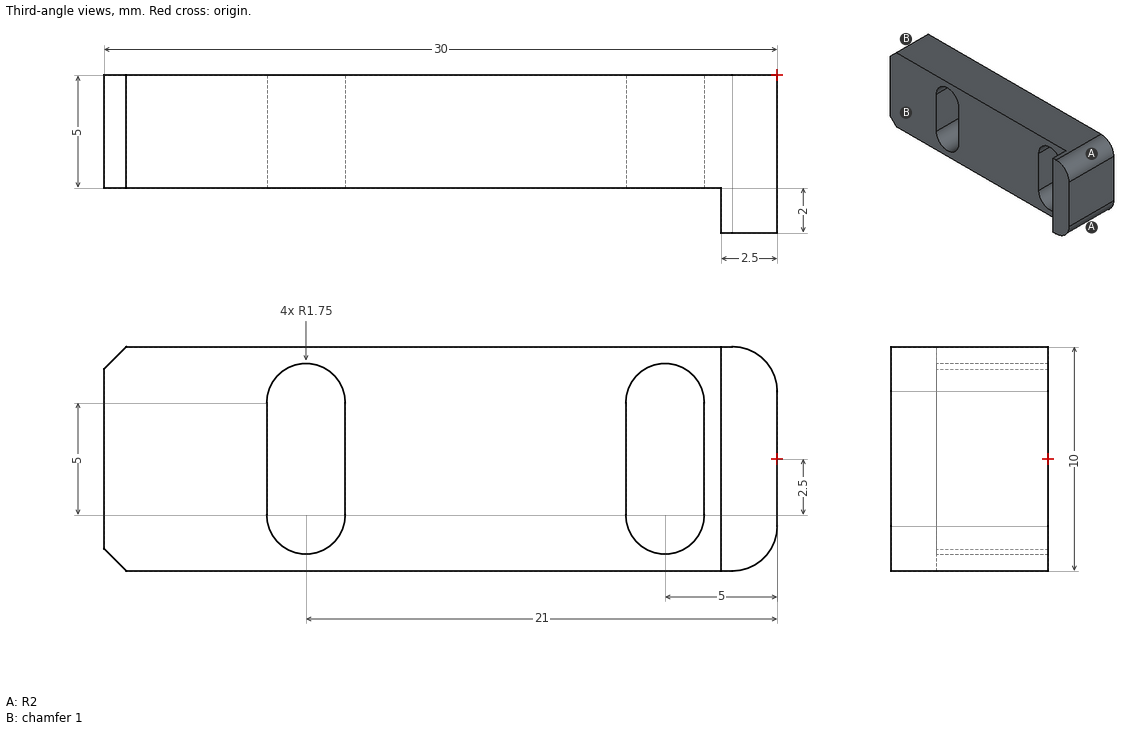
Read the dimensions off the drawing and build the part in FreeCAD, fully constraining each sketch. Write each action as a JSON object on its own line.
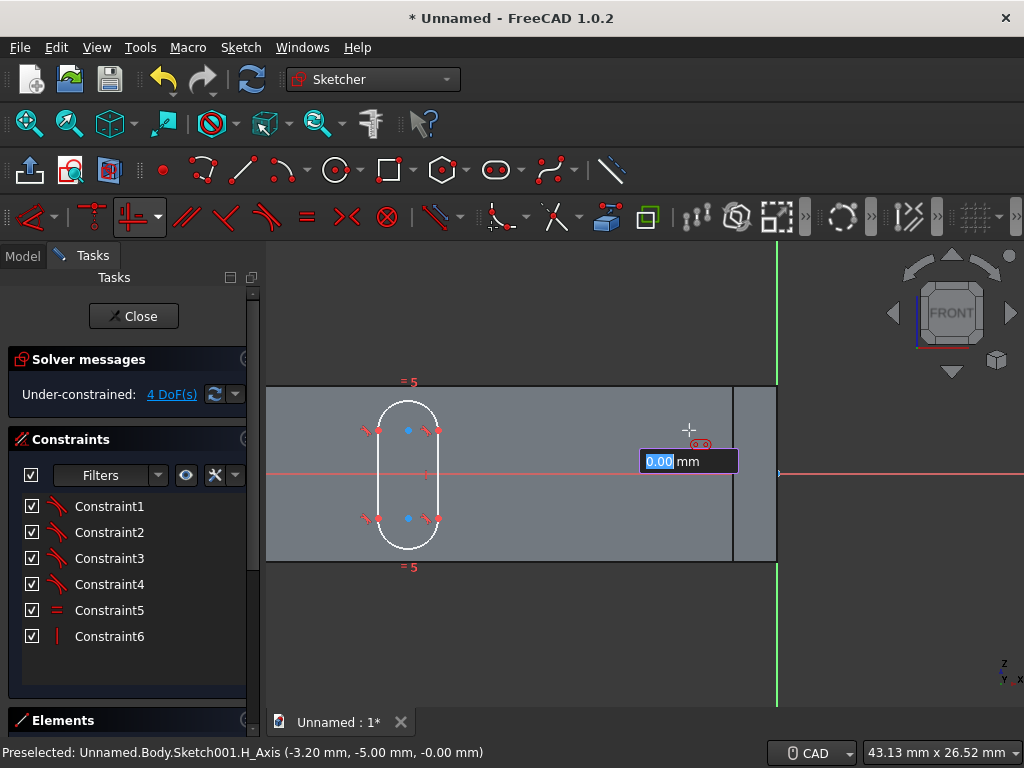
{"action": "left_click", "coordinate": [719, 487]}
{"action": "key", "text": "Escape"}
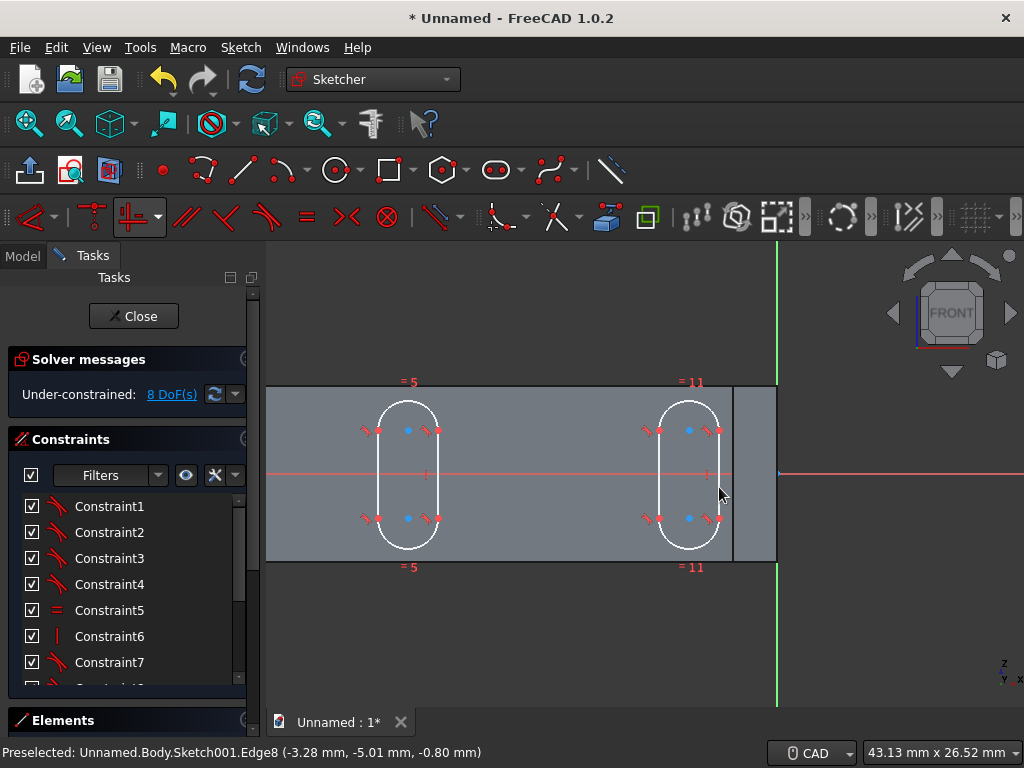
{"action": "left_click", "coordinate": [390, 543]}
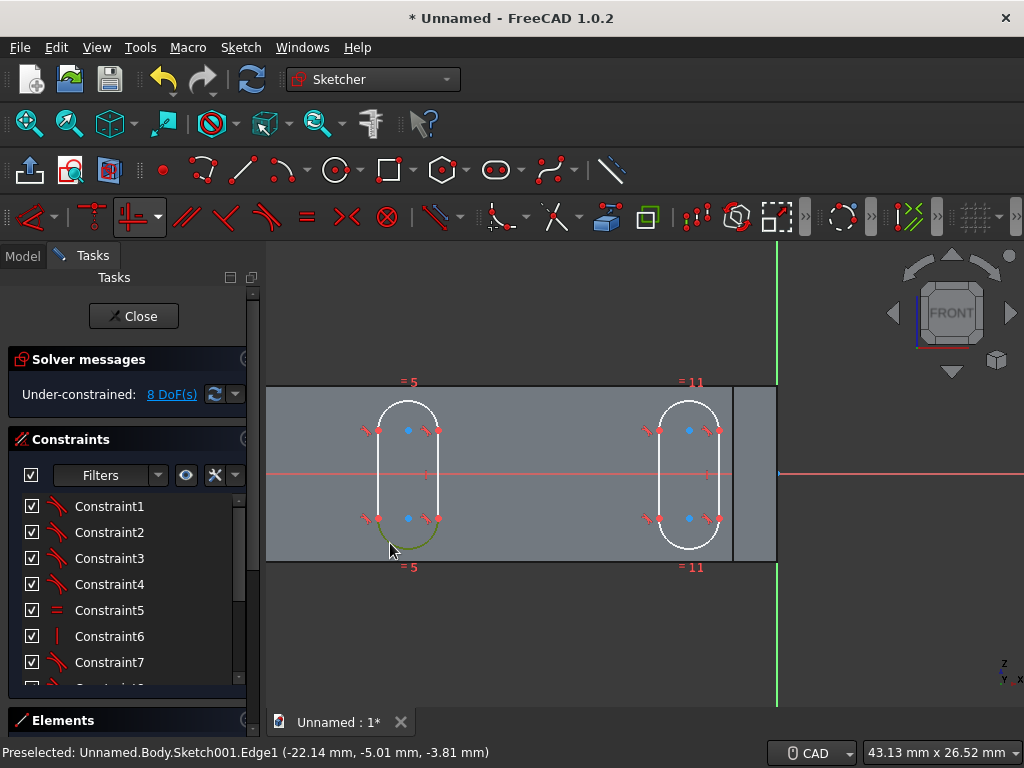
{"action": "left_click", "coordinate": [671, 543]}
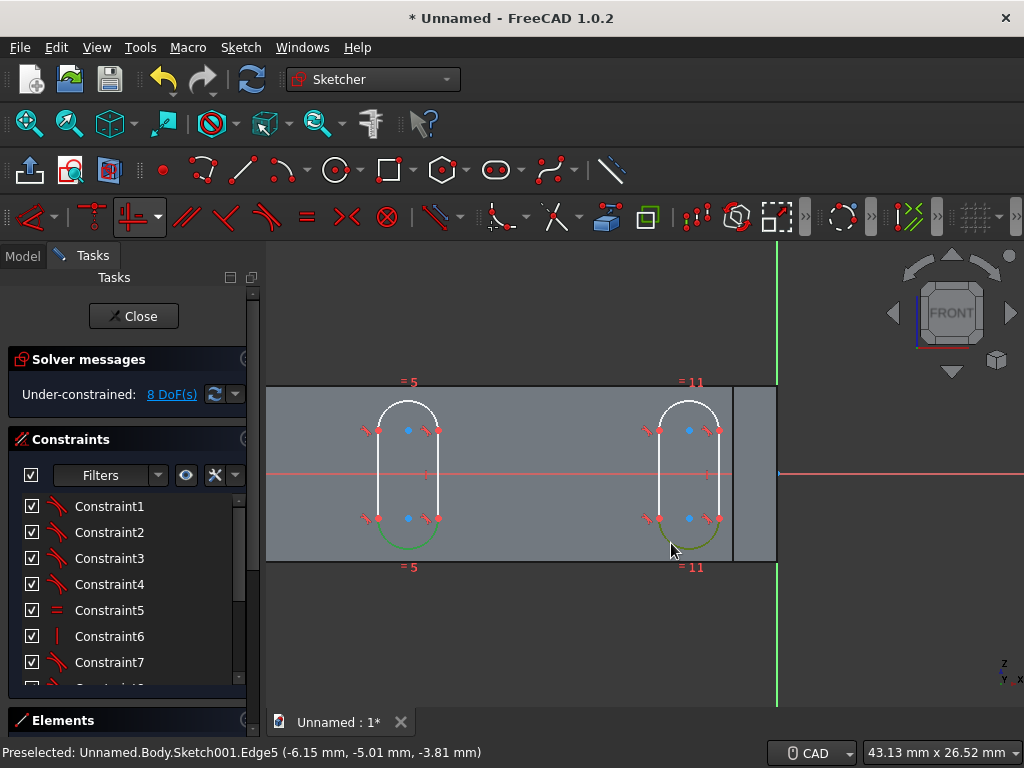
{"action": "left_click", "coordinate": [308, 218]}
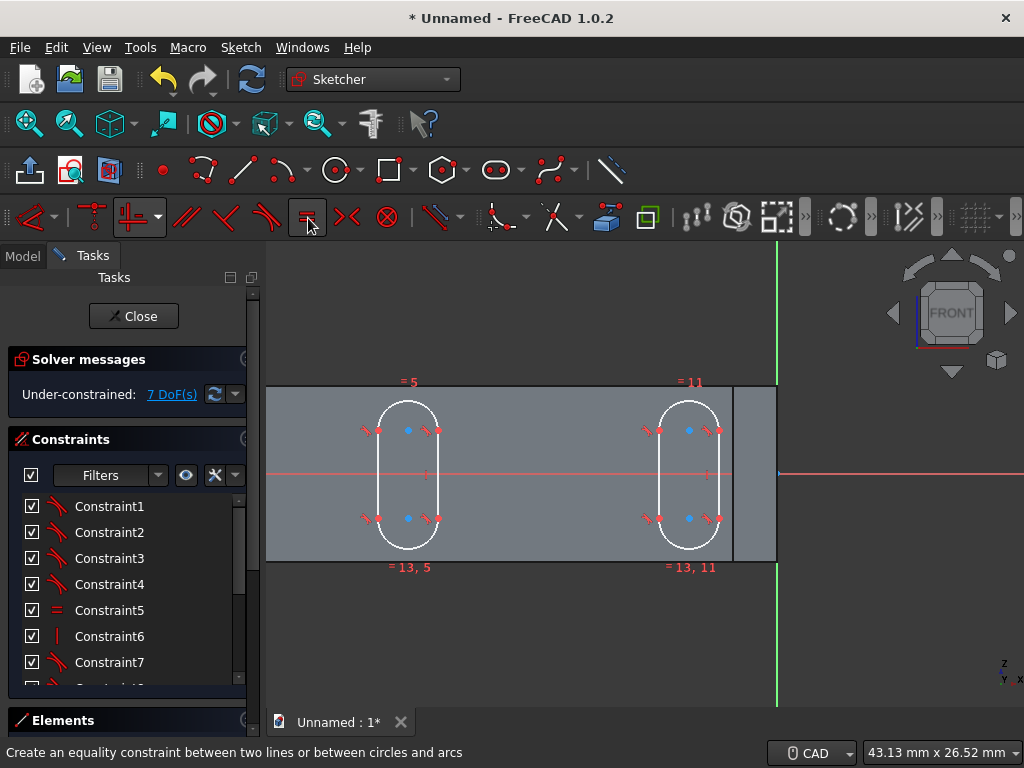
{"action": "scroll", "coordinate": [390, 543], "scroll_direction": "up", "scroll_amount": 2}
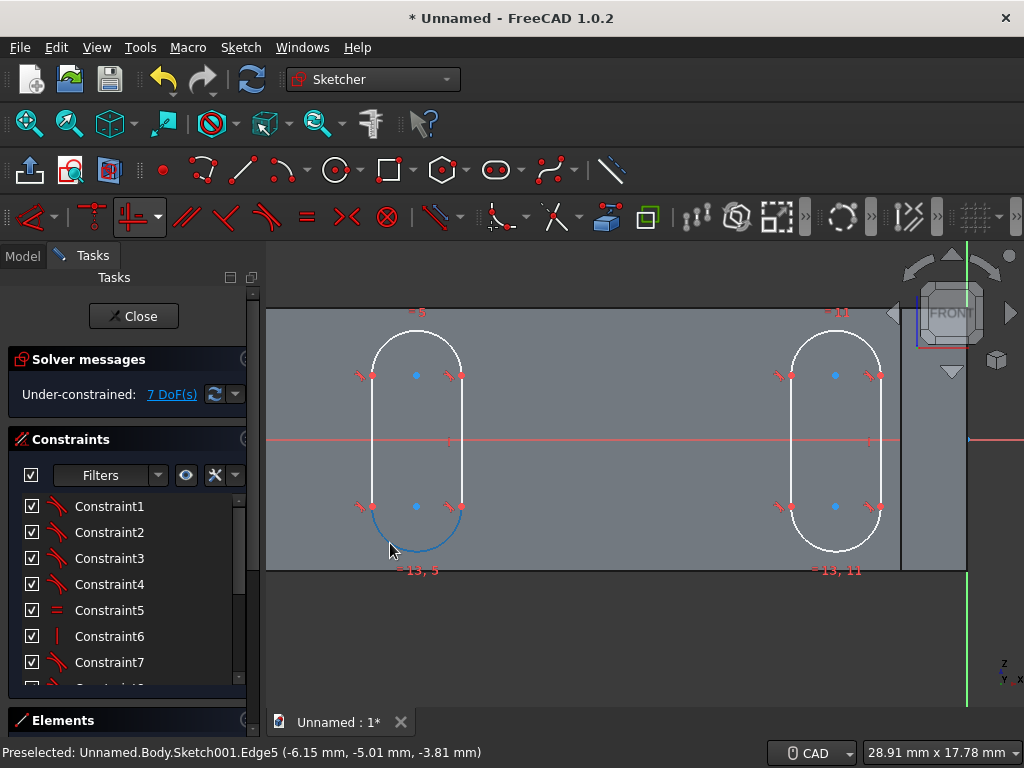
{"action": "left_click", "coordinate": [390, 543]}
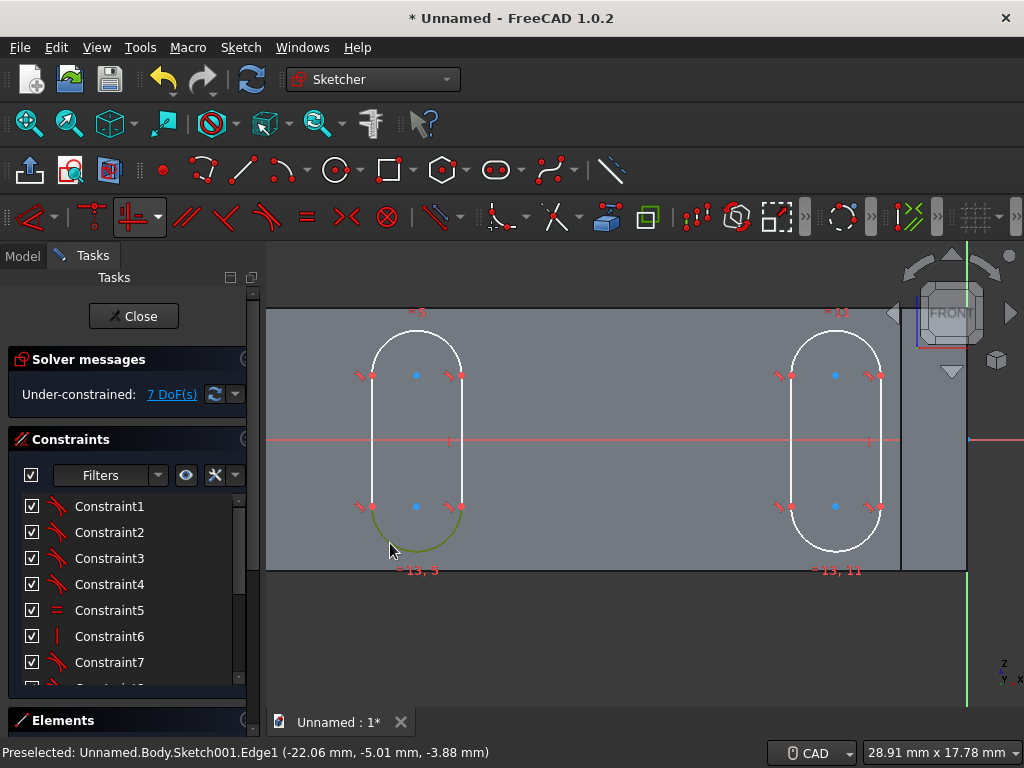
{"action": "key", "text": "k r"}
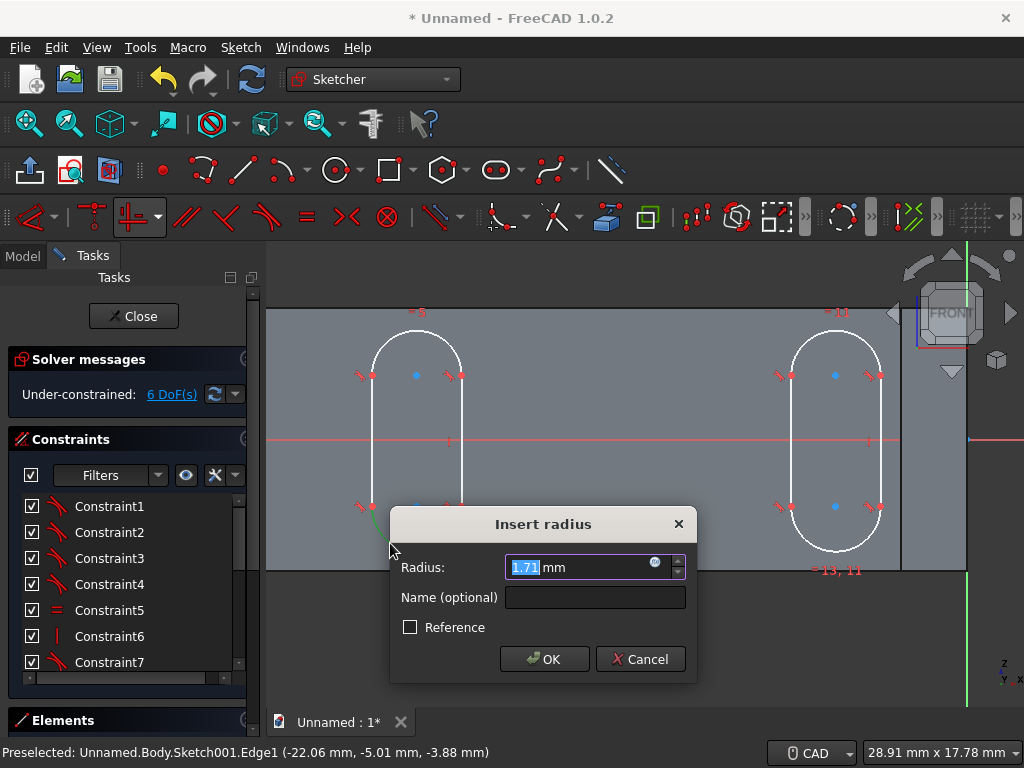
{"action": "type", "text": "1.75"}
{"action": "key", "text": "Return"}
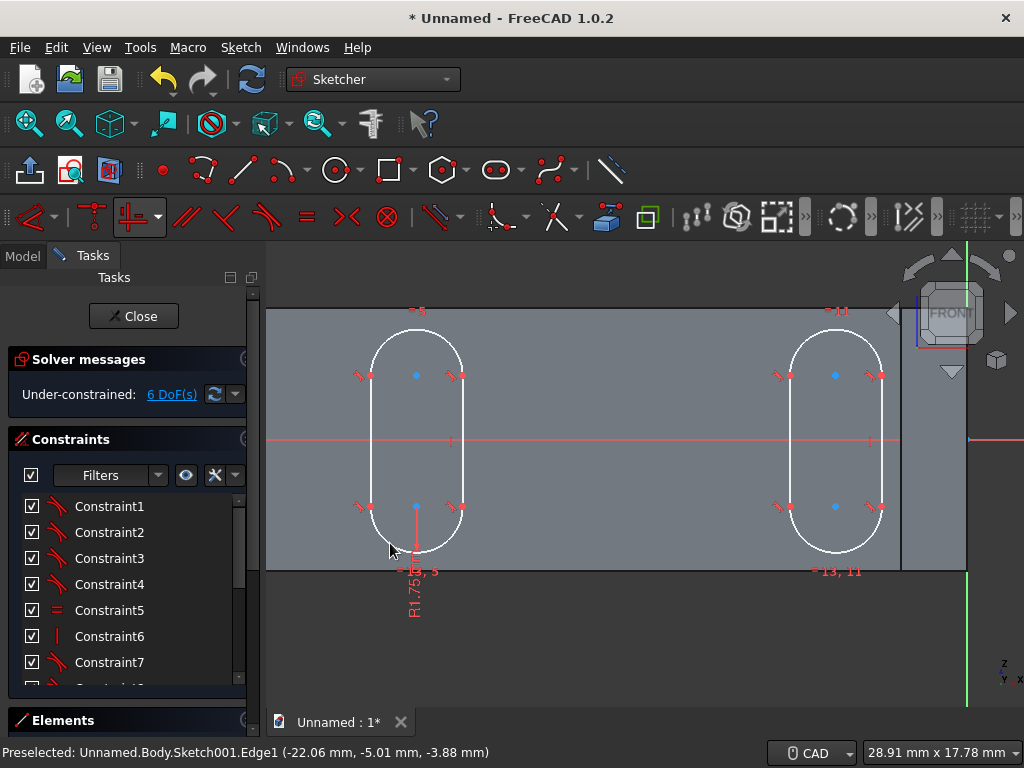
{"action": "left_click", "coordinate": [371, 467]}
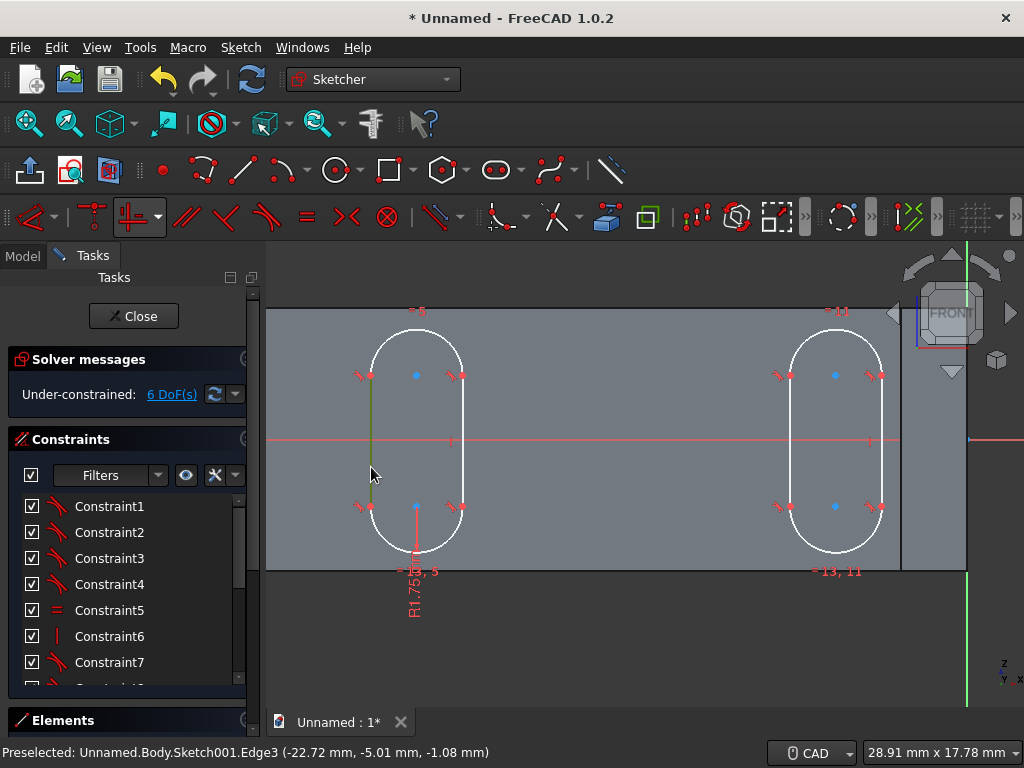
{"action": "key", "text": "i"}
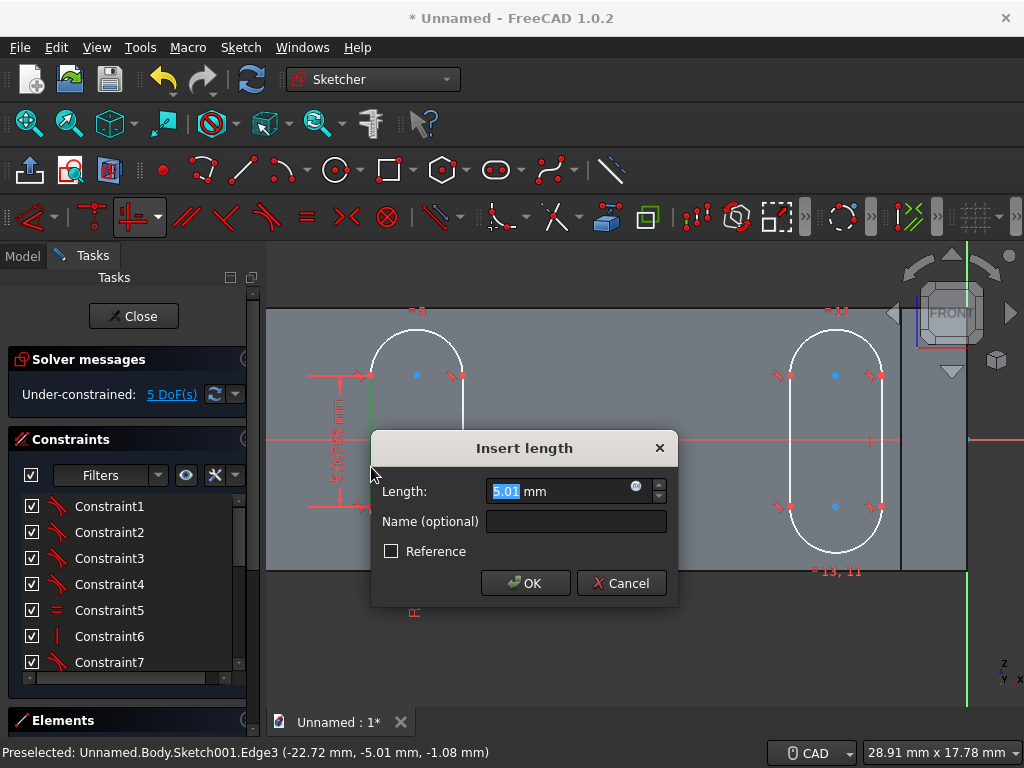
{"action": "type", "text": "5"}
{"action": "key", "text": "Return"}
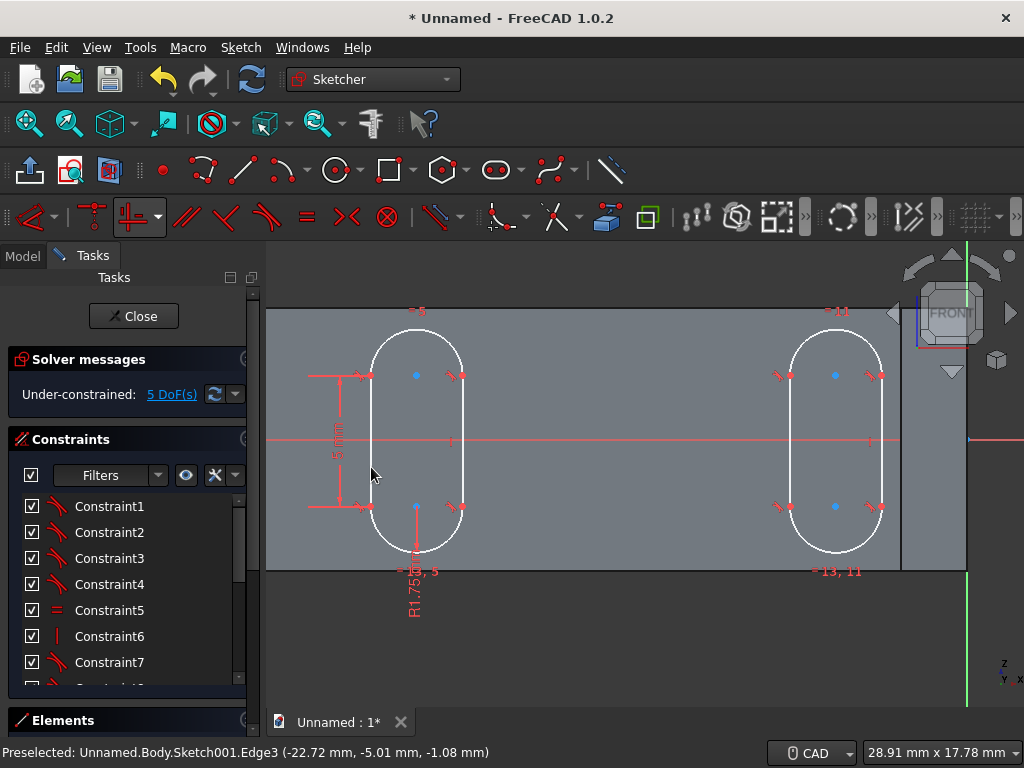
{"action": "left_click", "coordinate": [790, 467]}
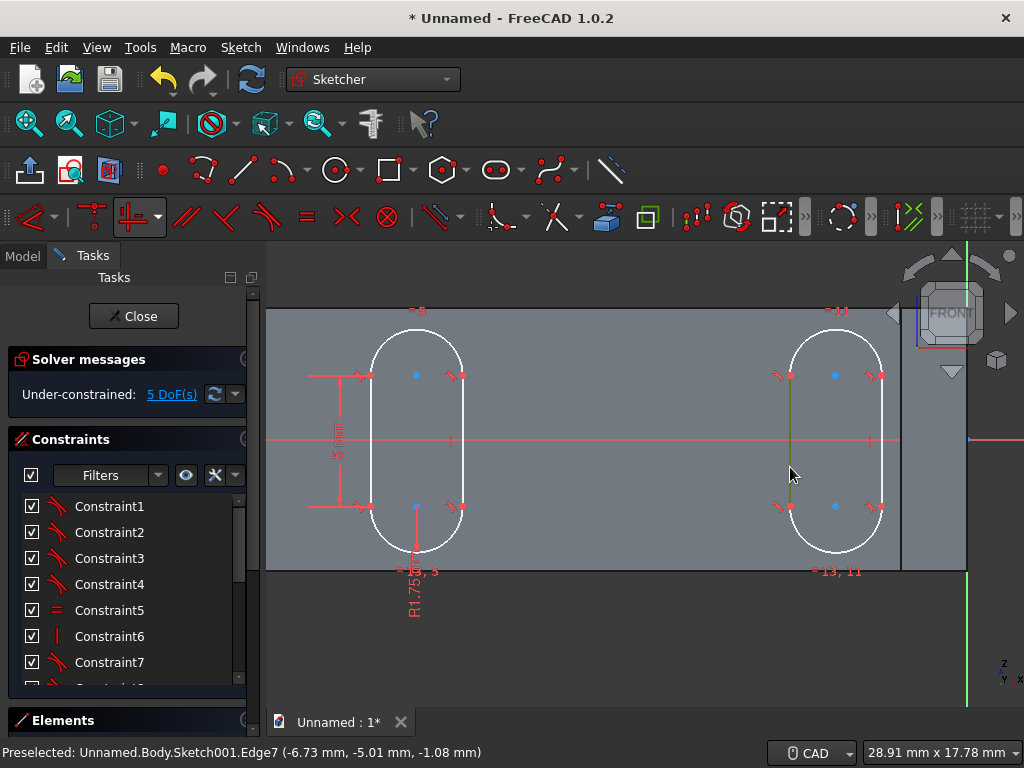
{"action": "key", "text": "i"}